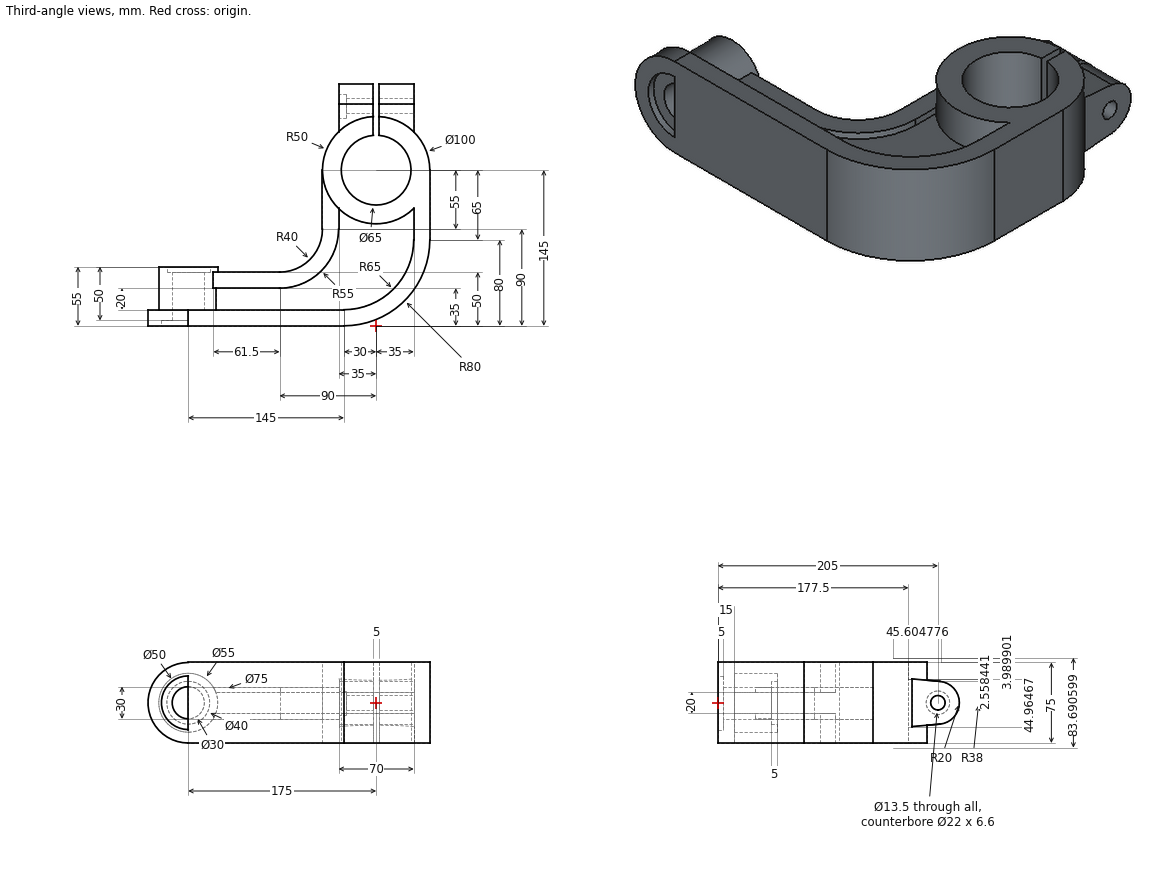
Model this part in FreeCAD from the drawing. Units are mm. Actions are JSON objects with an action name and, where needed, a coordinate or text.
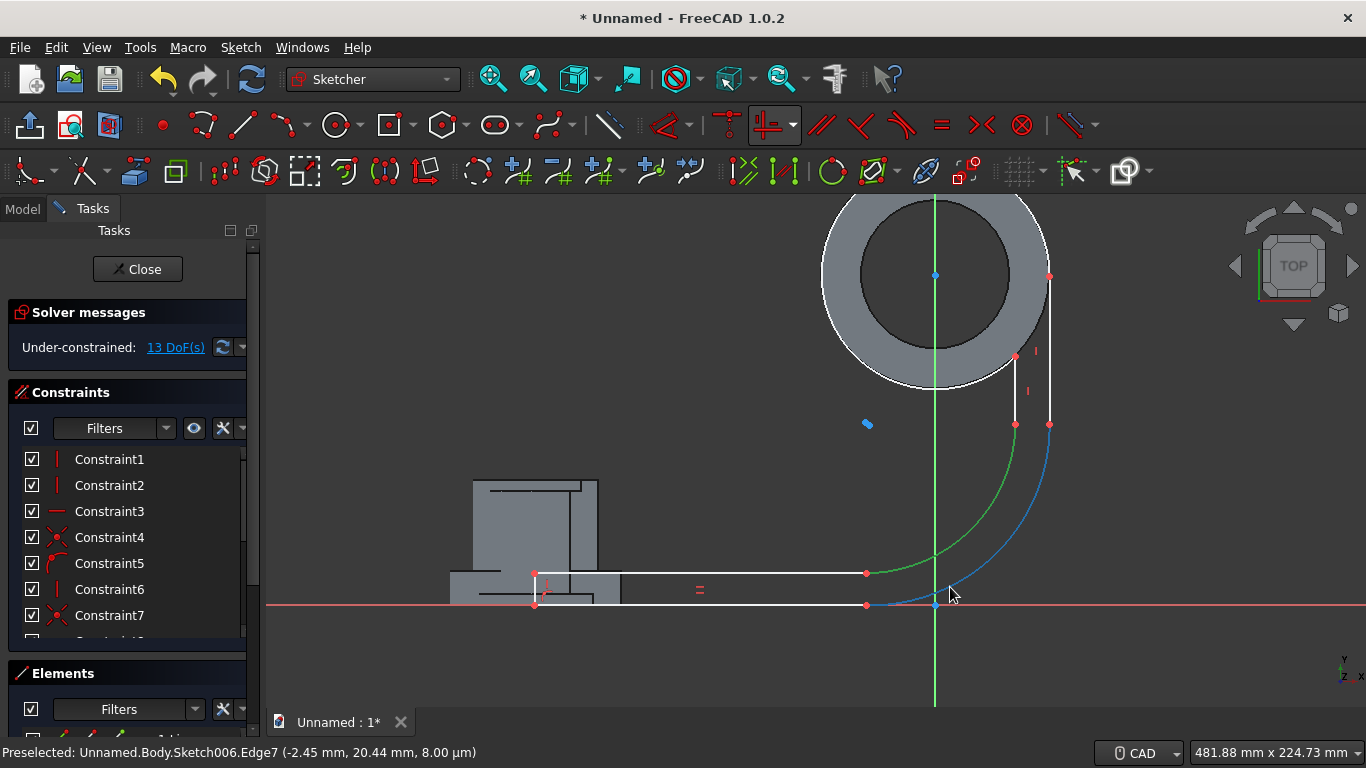
{"action": "left_click", "coordinate": [950, 587]}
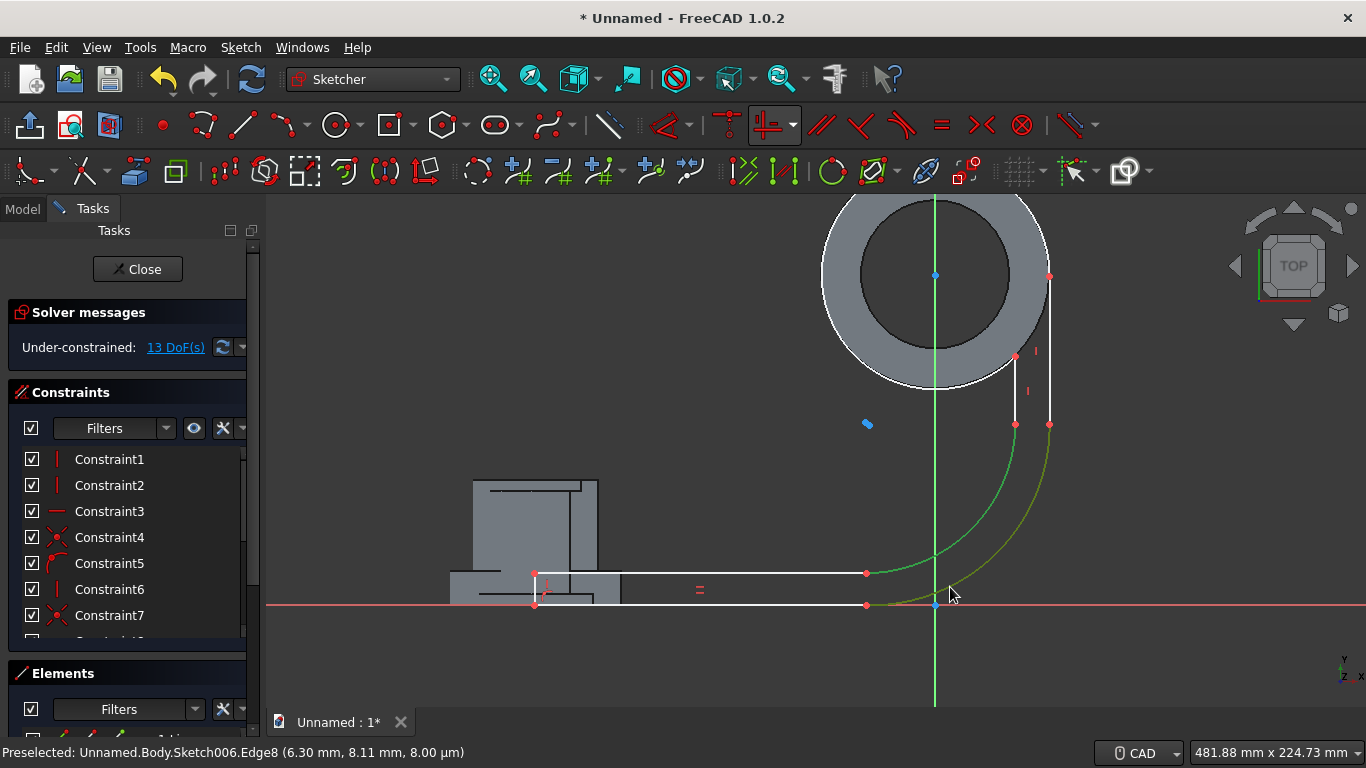
{"action": "left_click", "coordinate": [728, 126]}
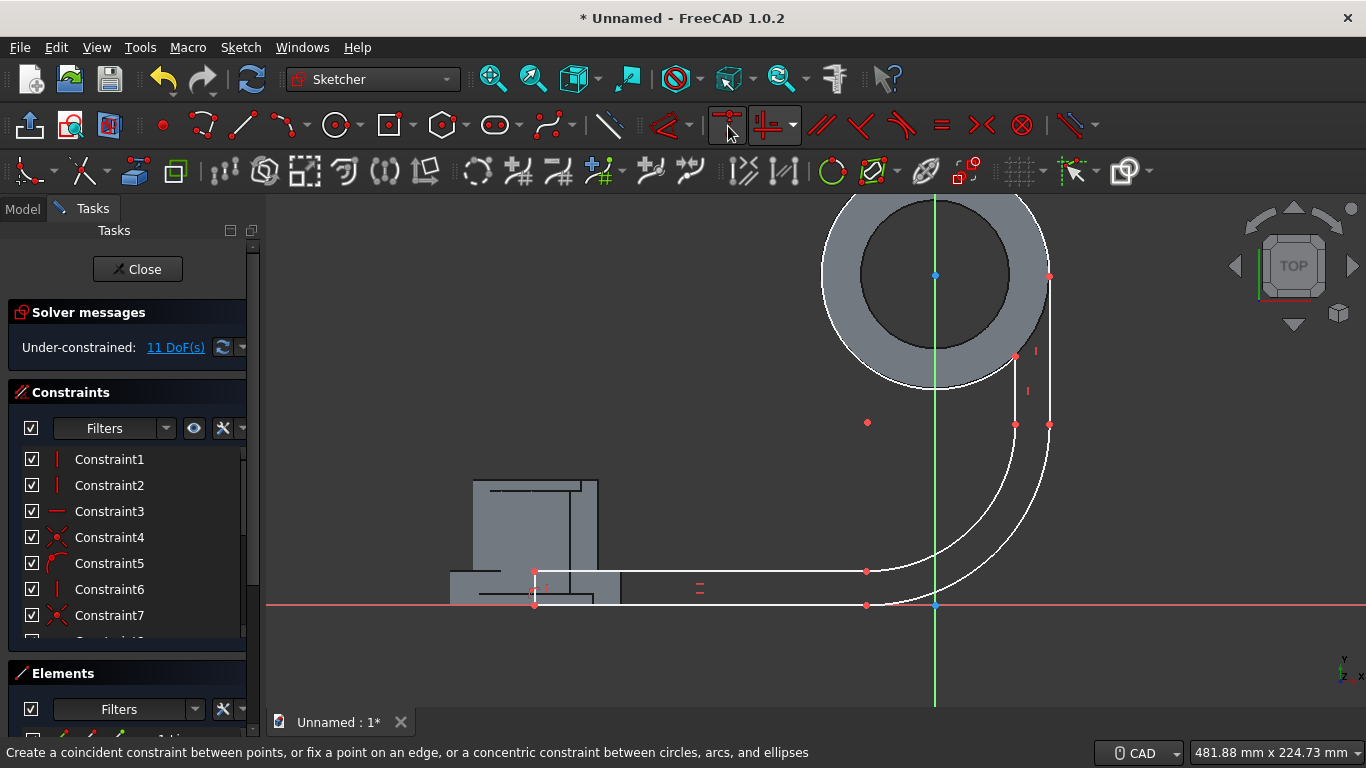
{"action": "left_click", "coordinate": [936, 275]}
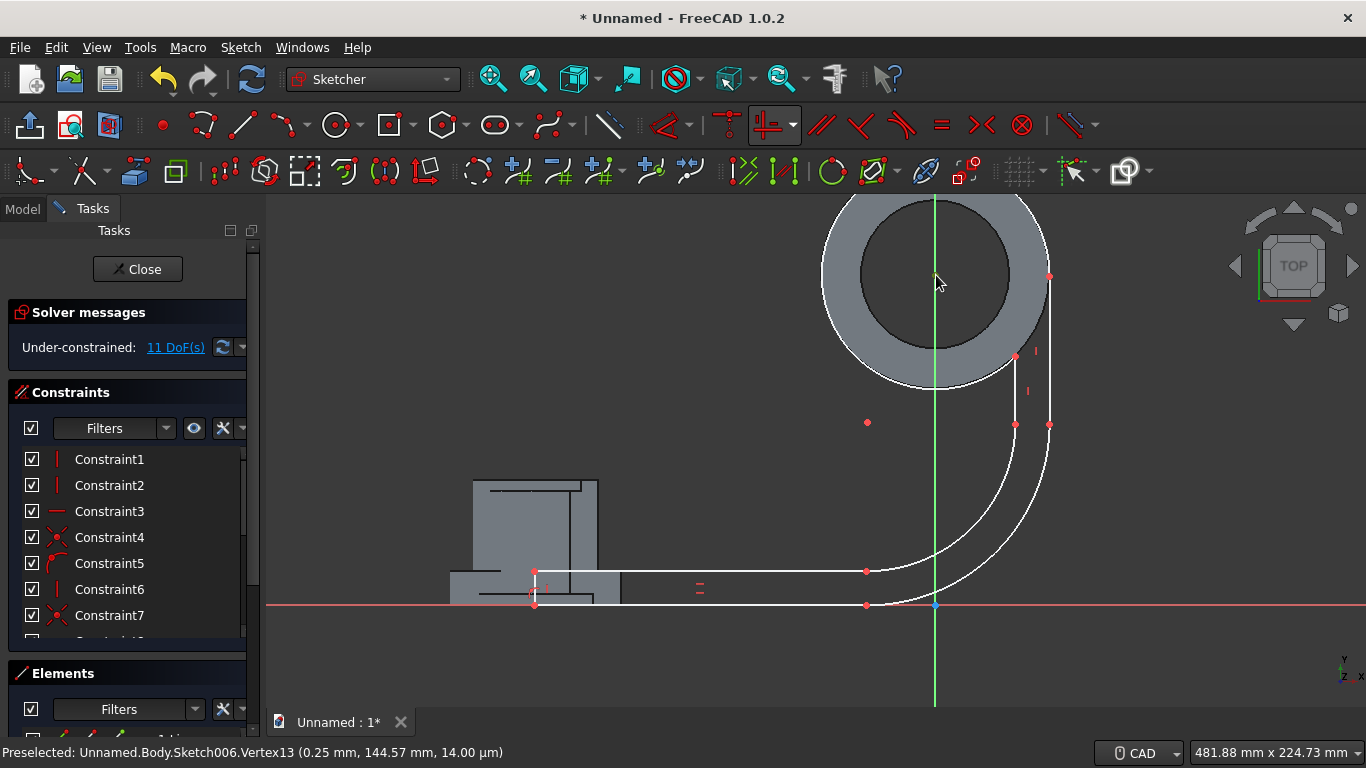
{"action": "left_click", "coordinate": [935, 646]}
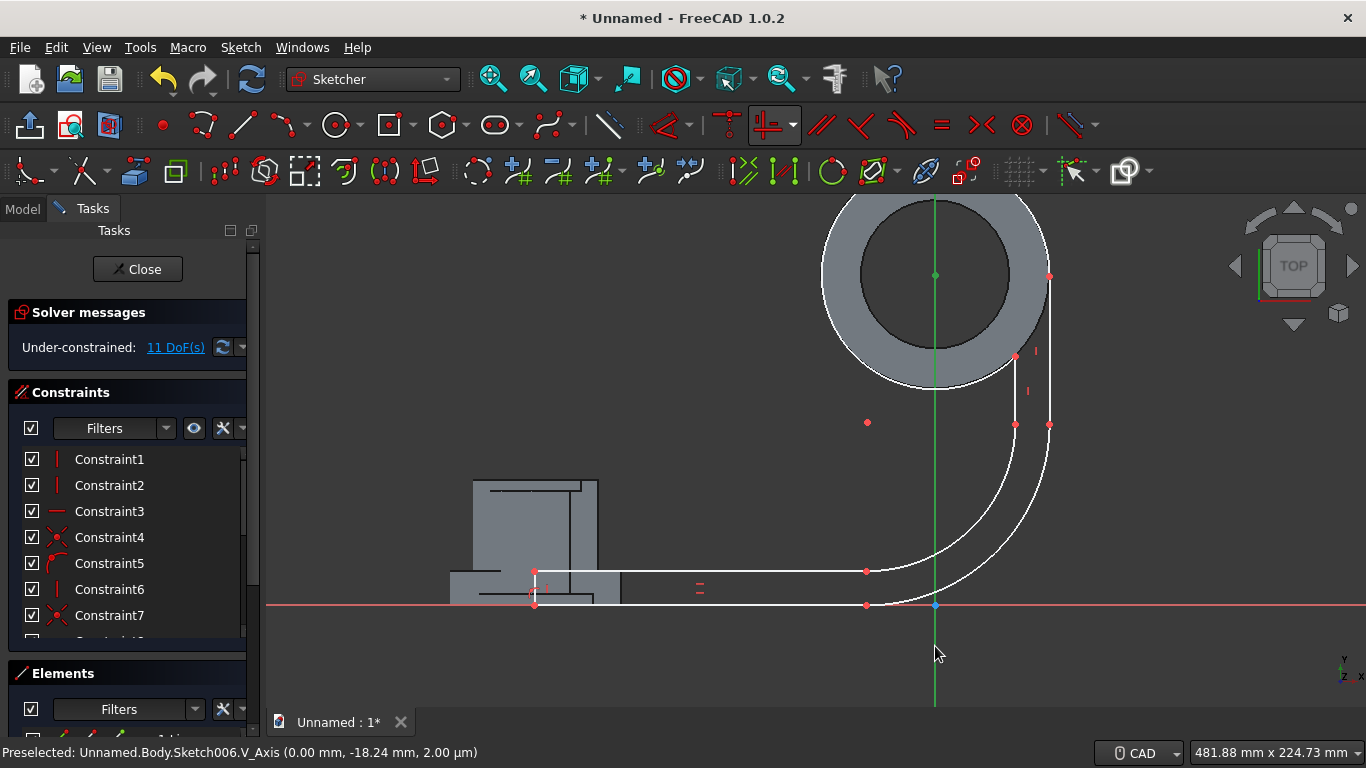
{"action": "key", "text": "c"}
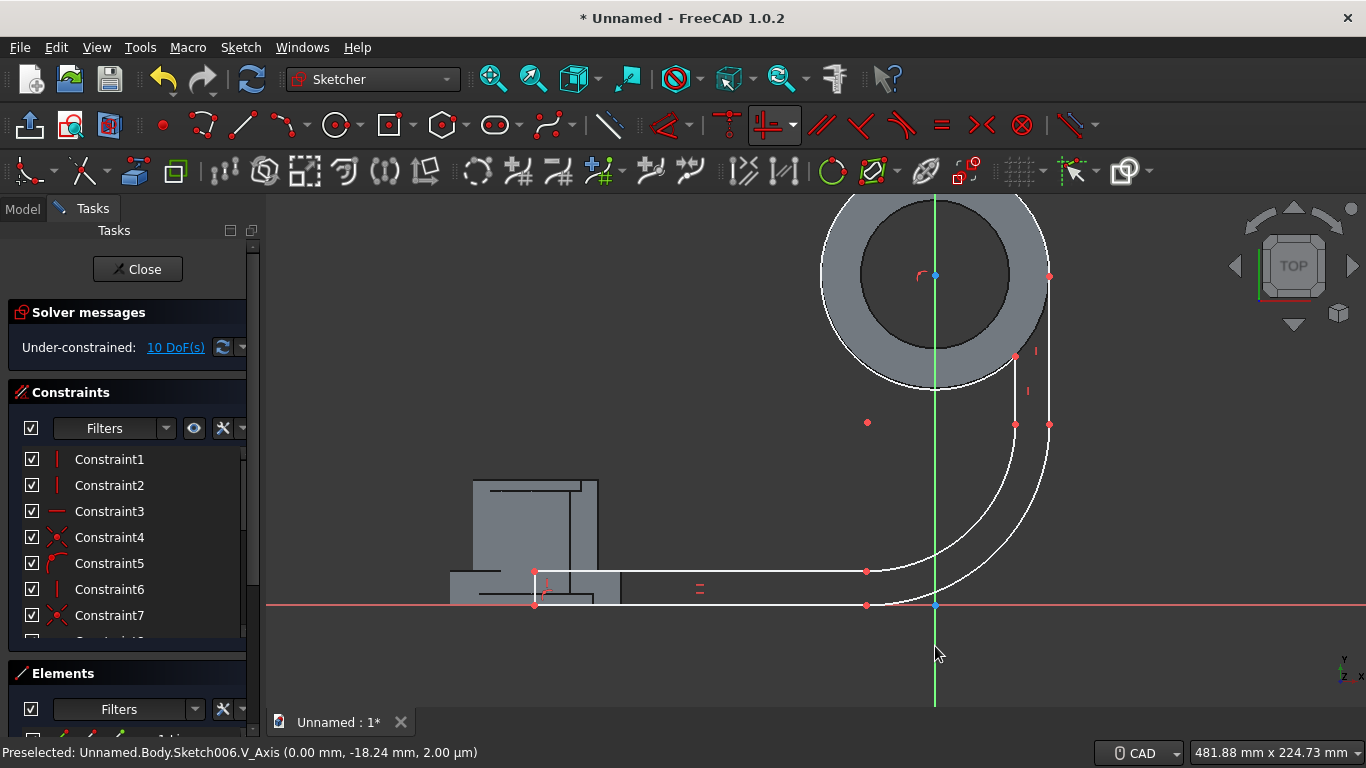
{"action": "left_click", "coordinate": [664, 126]}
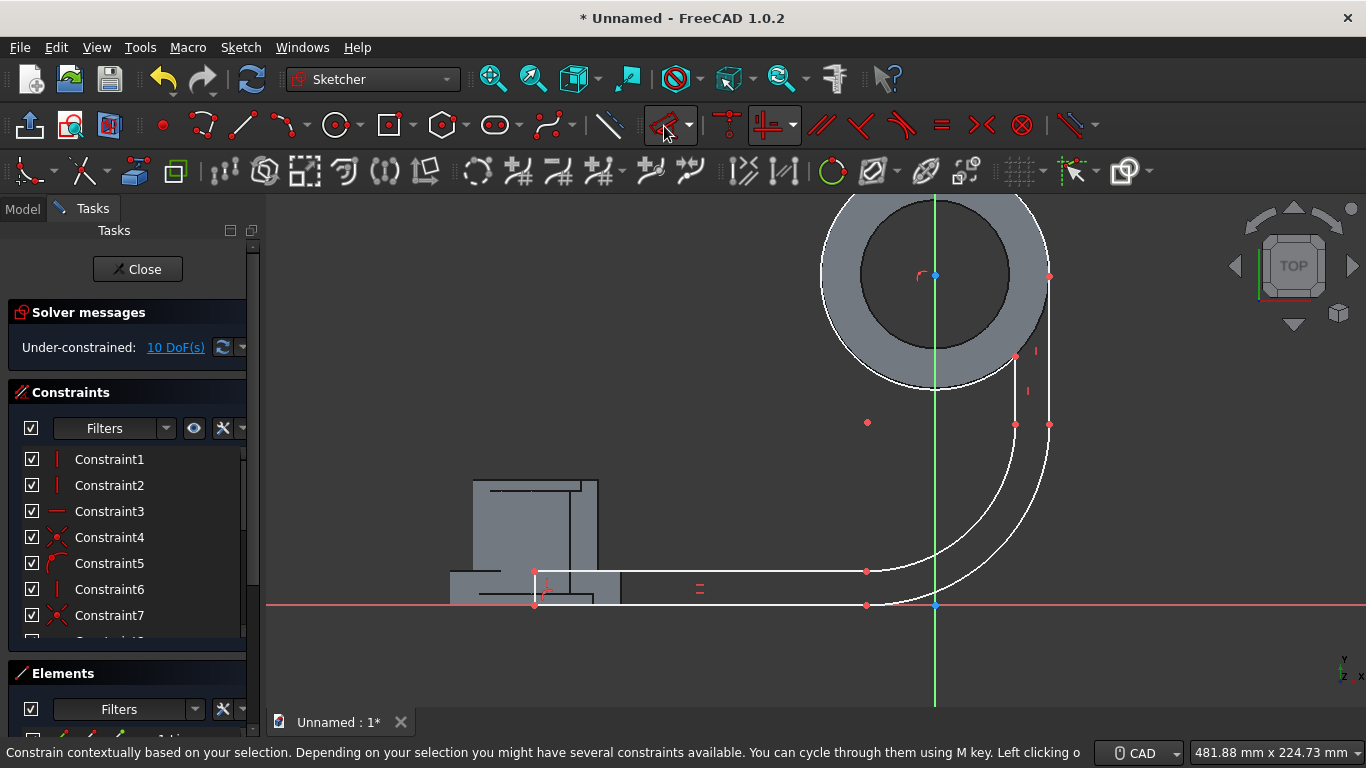
{"action": "left_click", "coordinate": [848, 349]}
{"action": "left_click", "coordinate": [824, 370]}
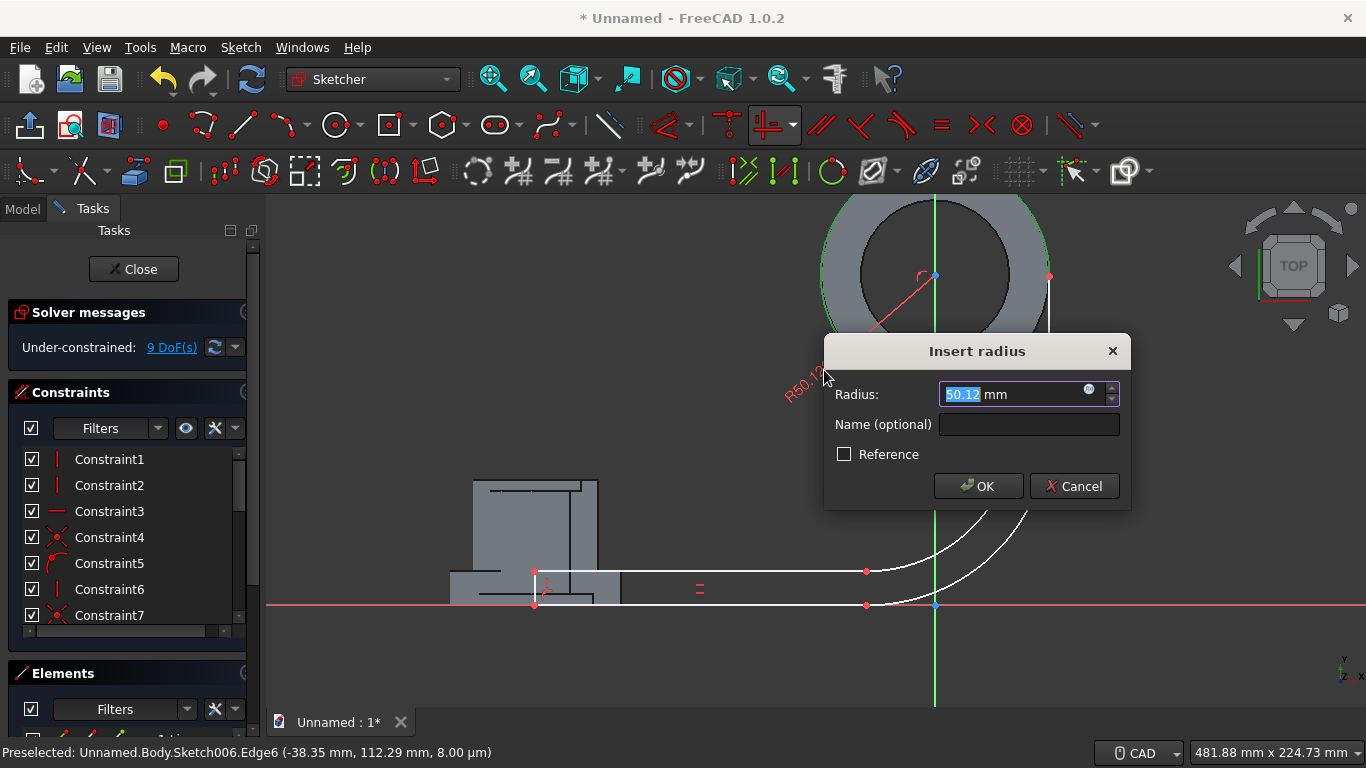
{"action": "type", "text": "50"}
{"action": "key", "text": "Return"}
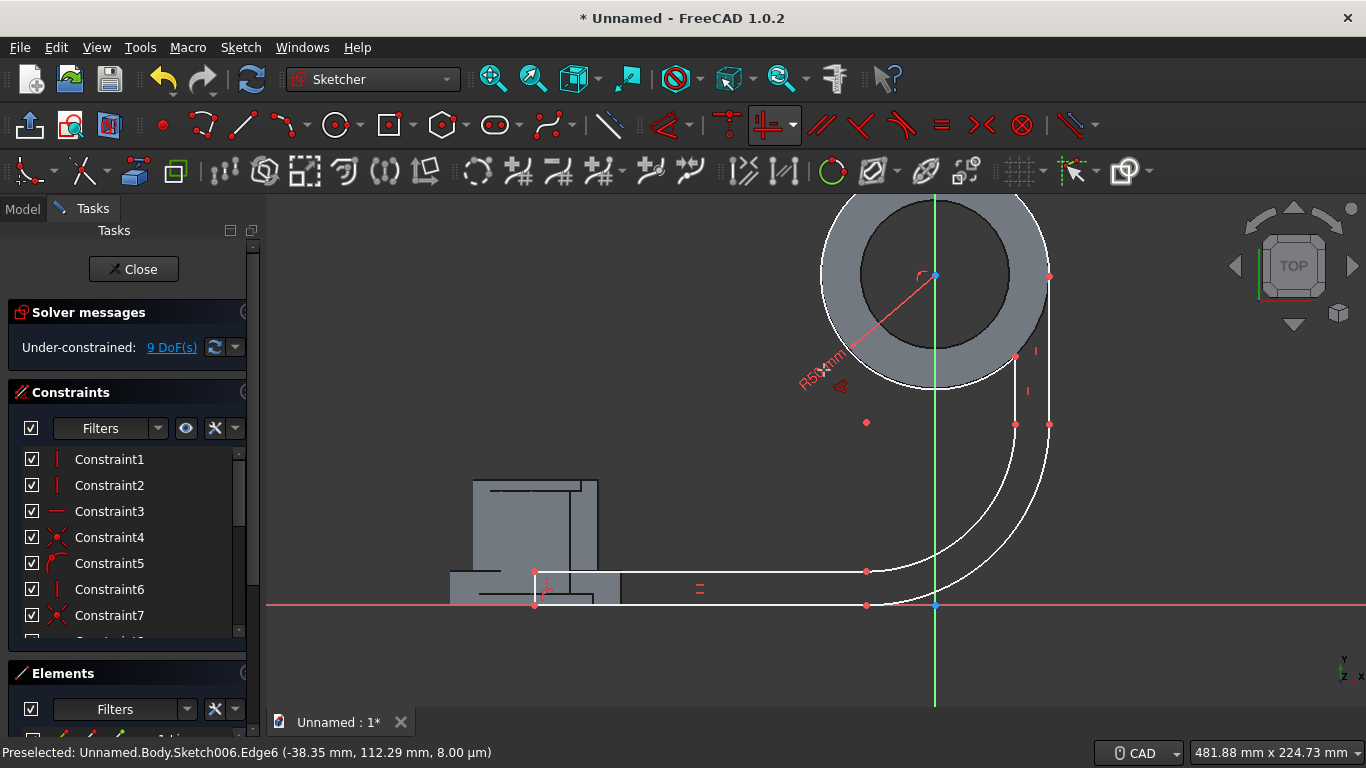
{"action": "left_click", "coordinate": [934, 556]}
{"action": "left_click", "coordinate": [705, 505]}